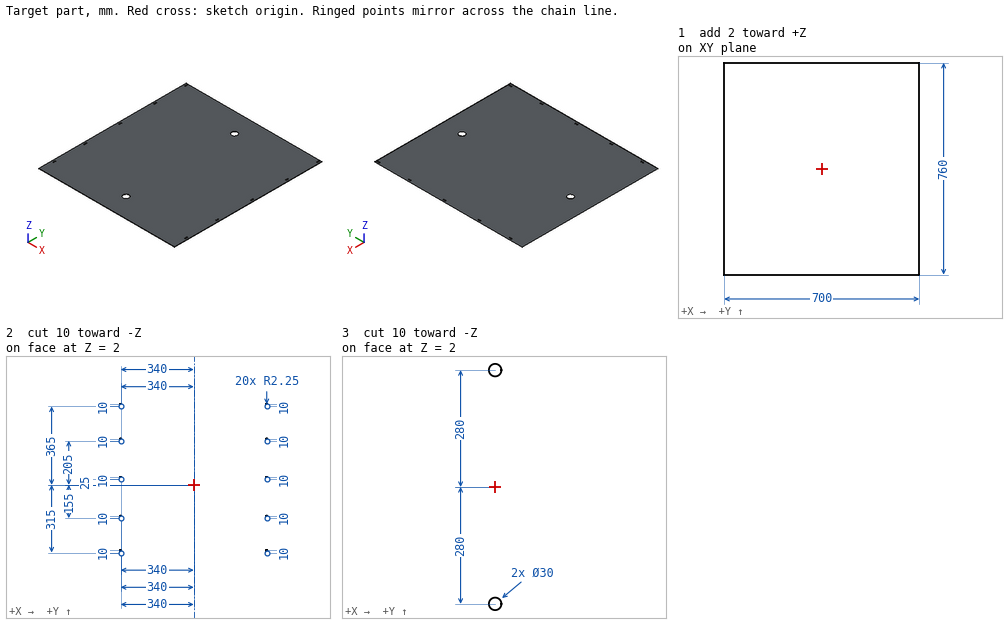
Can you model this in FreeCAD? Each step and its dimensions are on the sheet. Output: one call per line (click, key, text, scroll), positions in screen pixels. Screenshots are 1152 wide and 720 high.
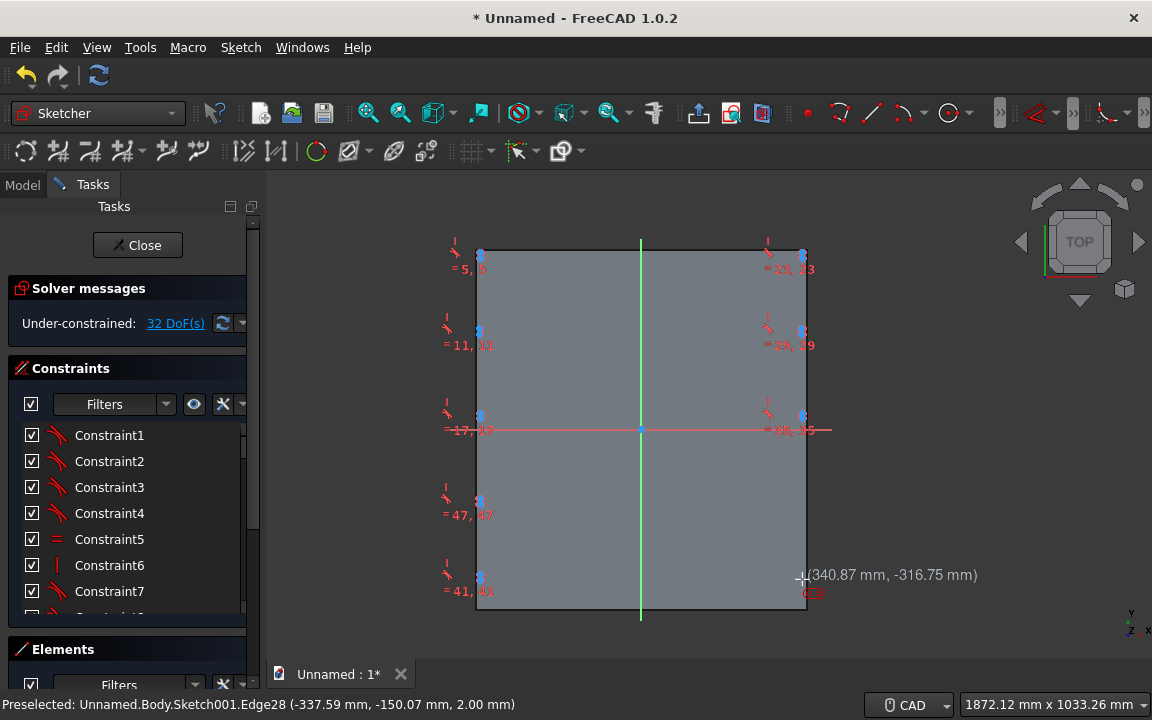
click(802, 579)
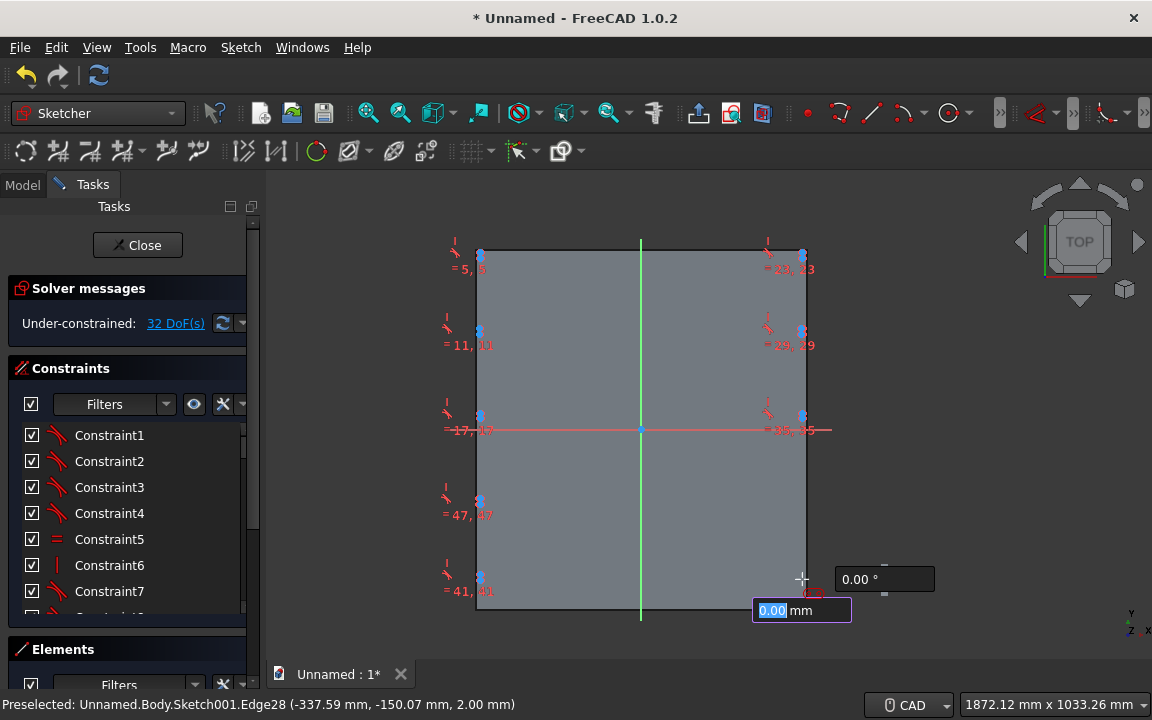
scroll(802, 574, up, 7)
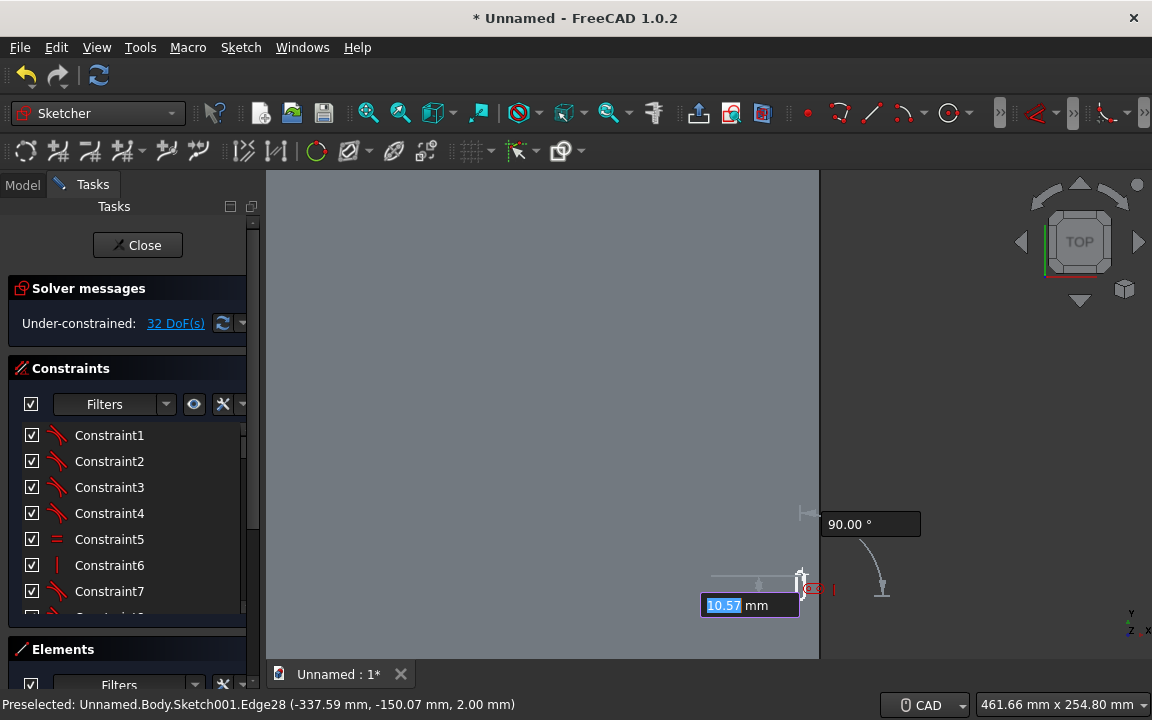
click(800, 573)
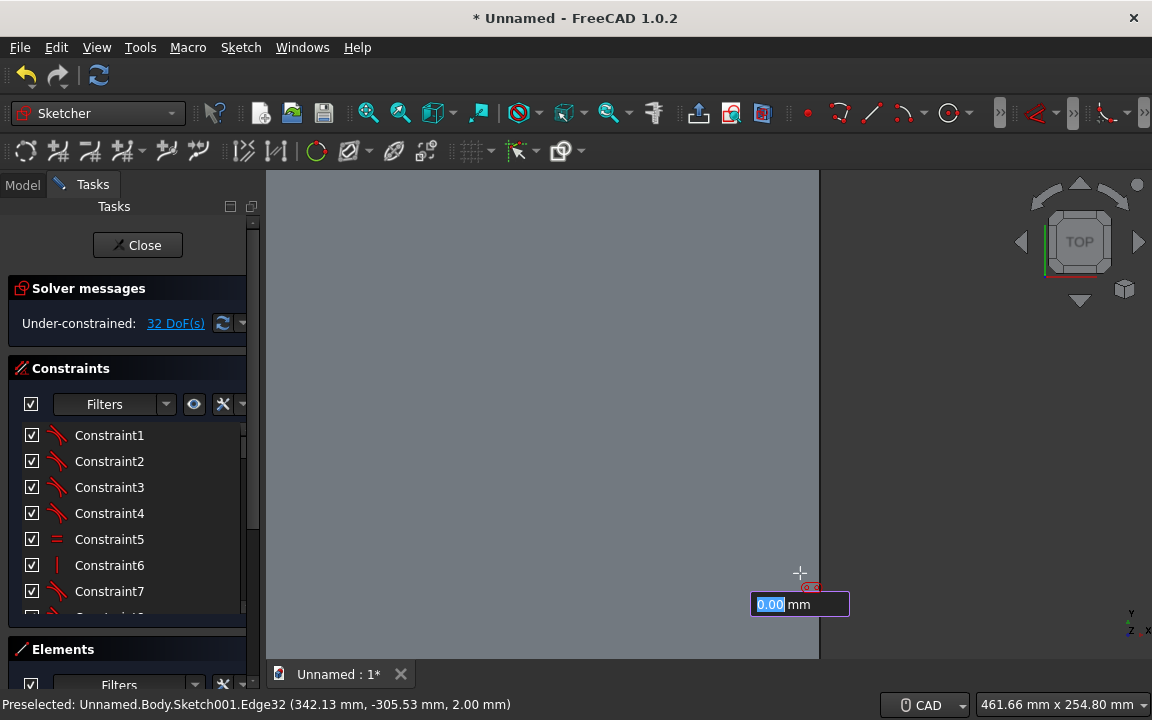
scroll(797, 582, up, 7)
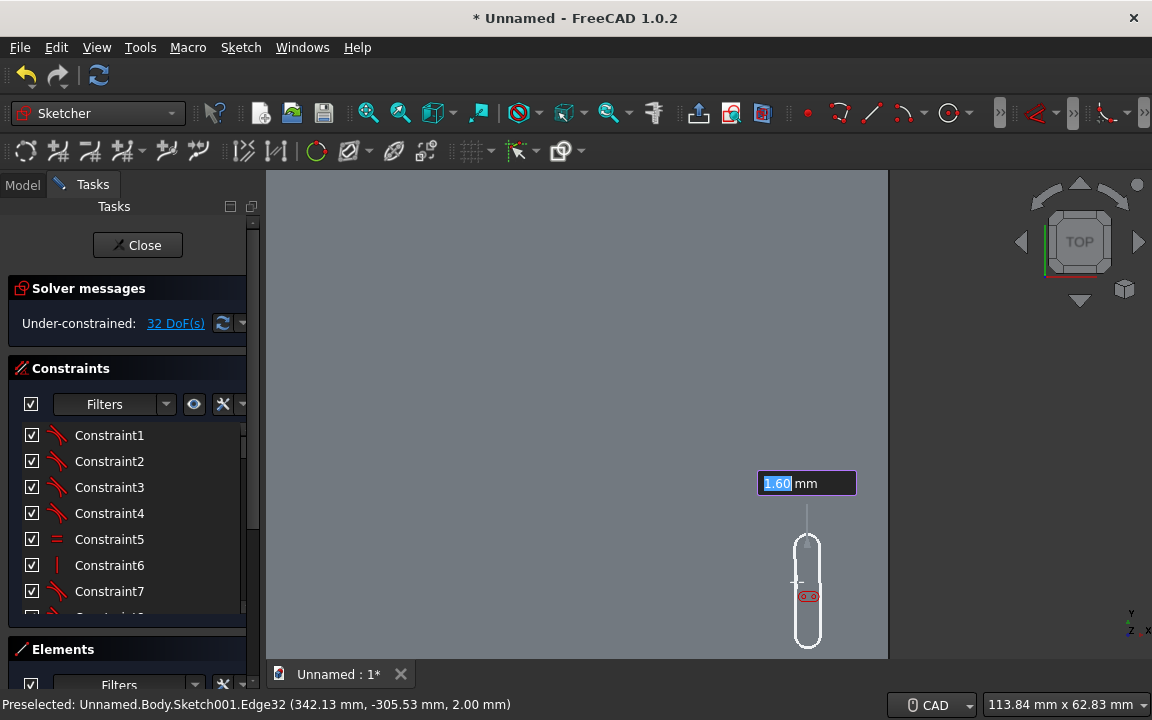
click(793, 580)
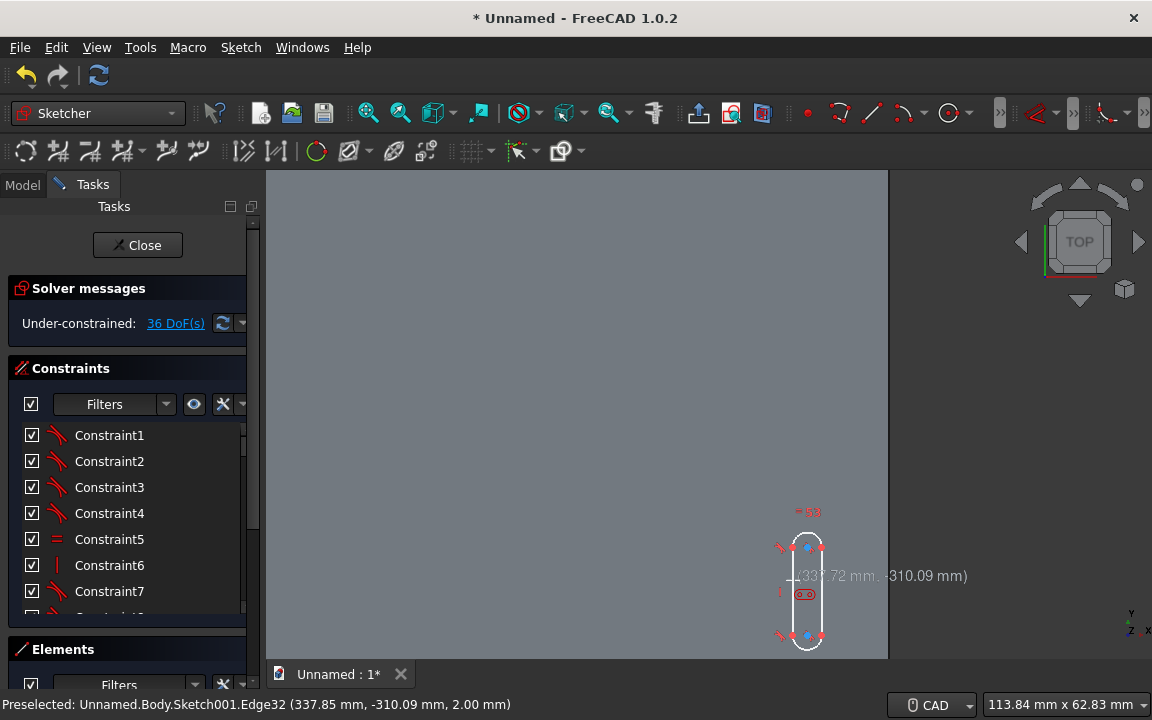
scroll(801, 575, down, 14)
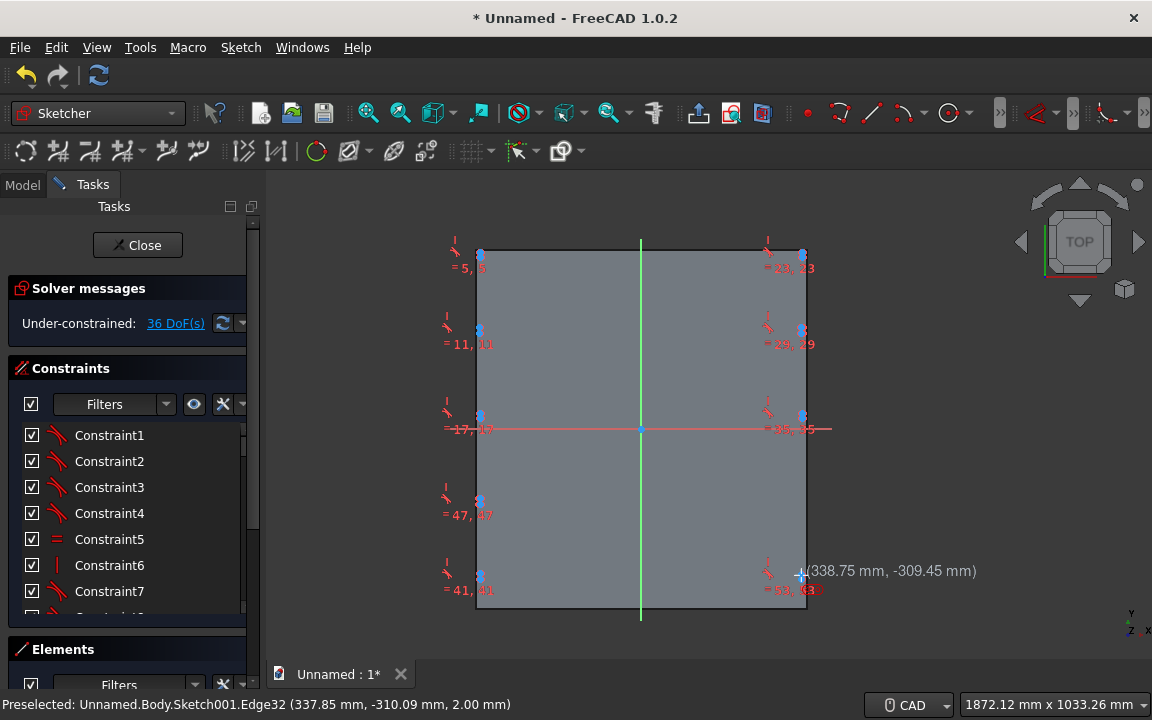
scroll(802, 503, up, 16)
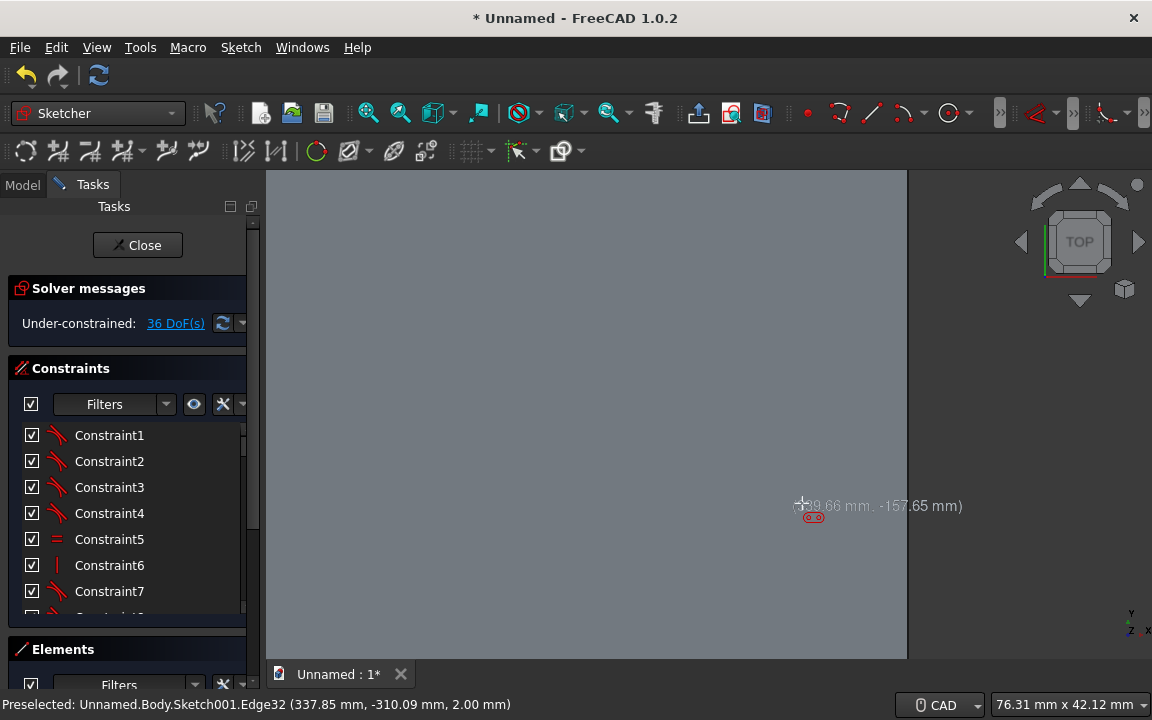
scroll(802, 503, down, 16)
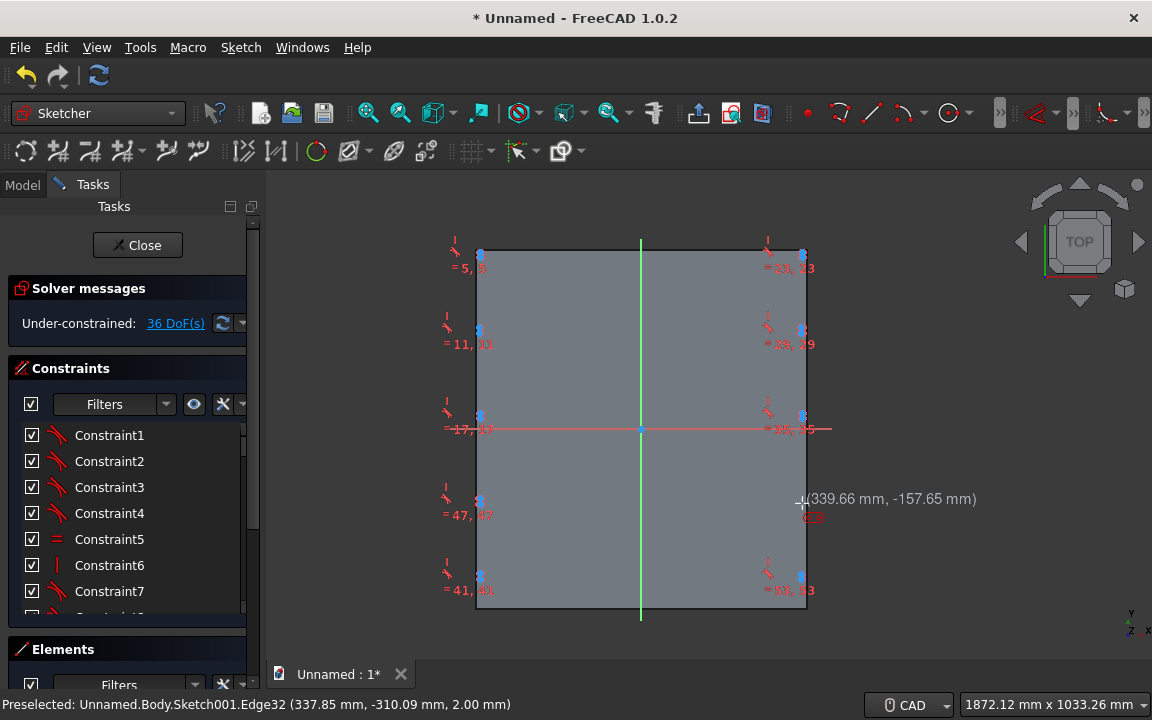
click(802, 503)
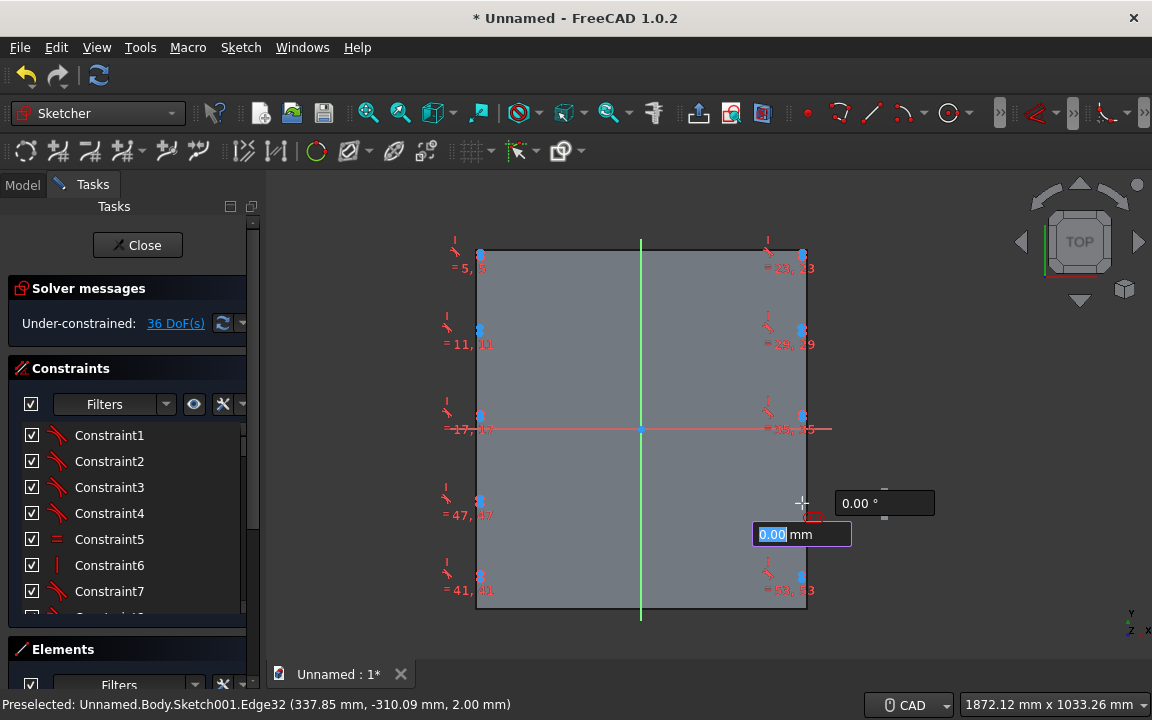
scroll(802, 498, up, 7)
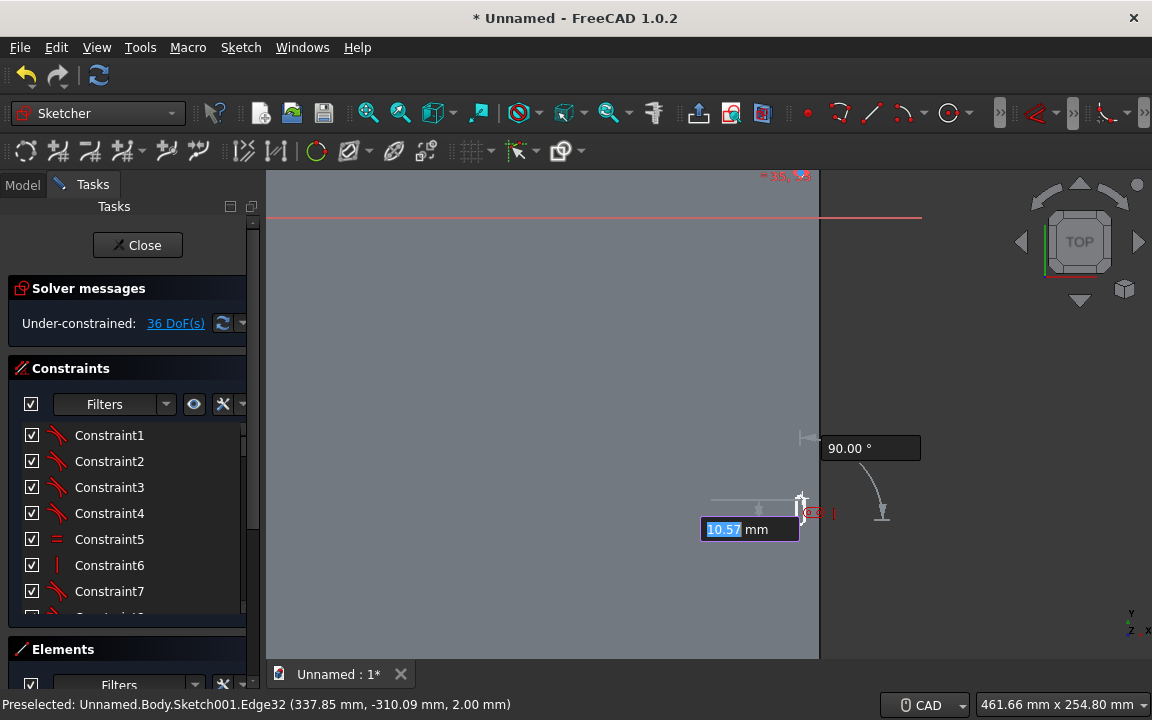
click(800, 496)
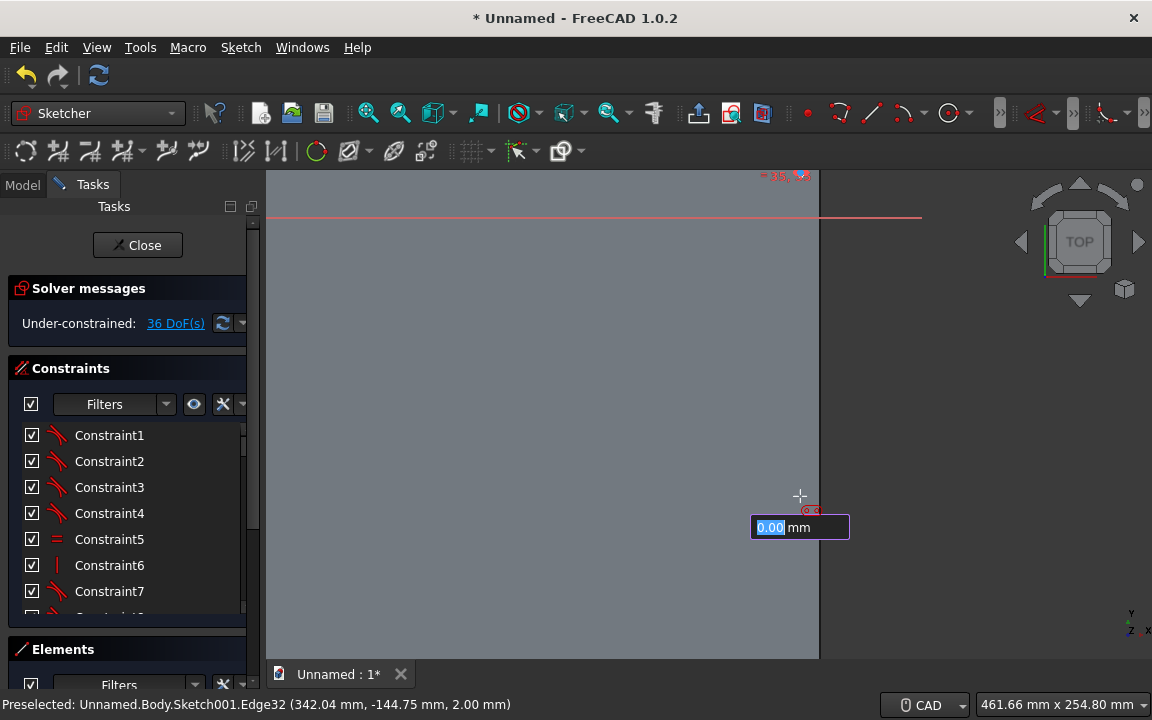
scroll(805, 506, up, 7)